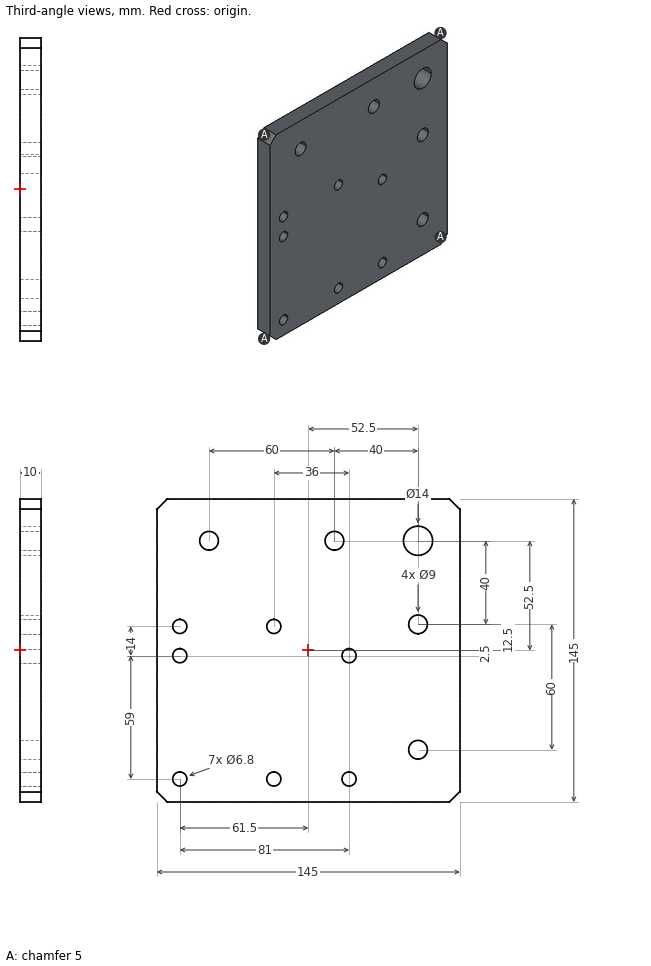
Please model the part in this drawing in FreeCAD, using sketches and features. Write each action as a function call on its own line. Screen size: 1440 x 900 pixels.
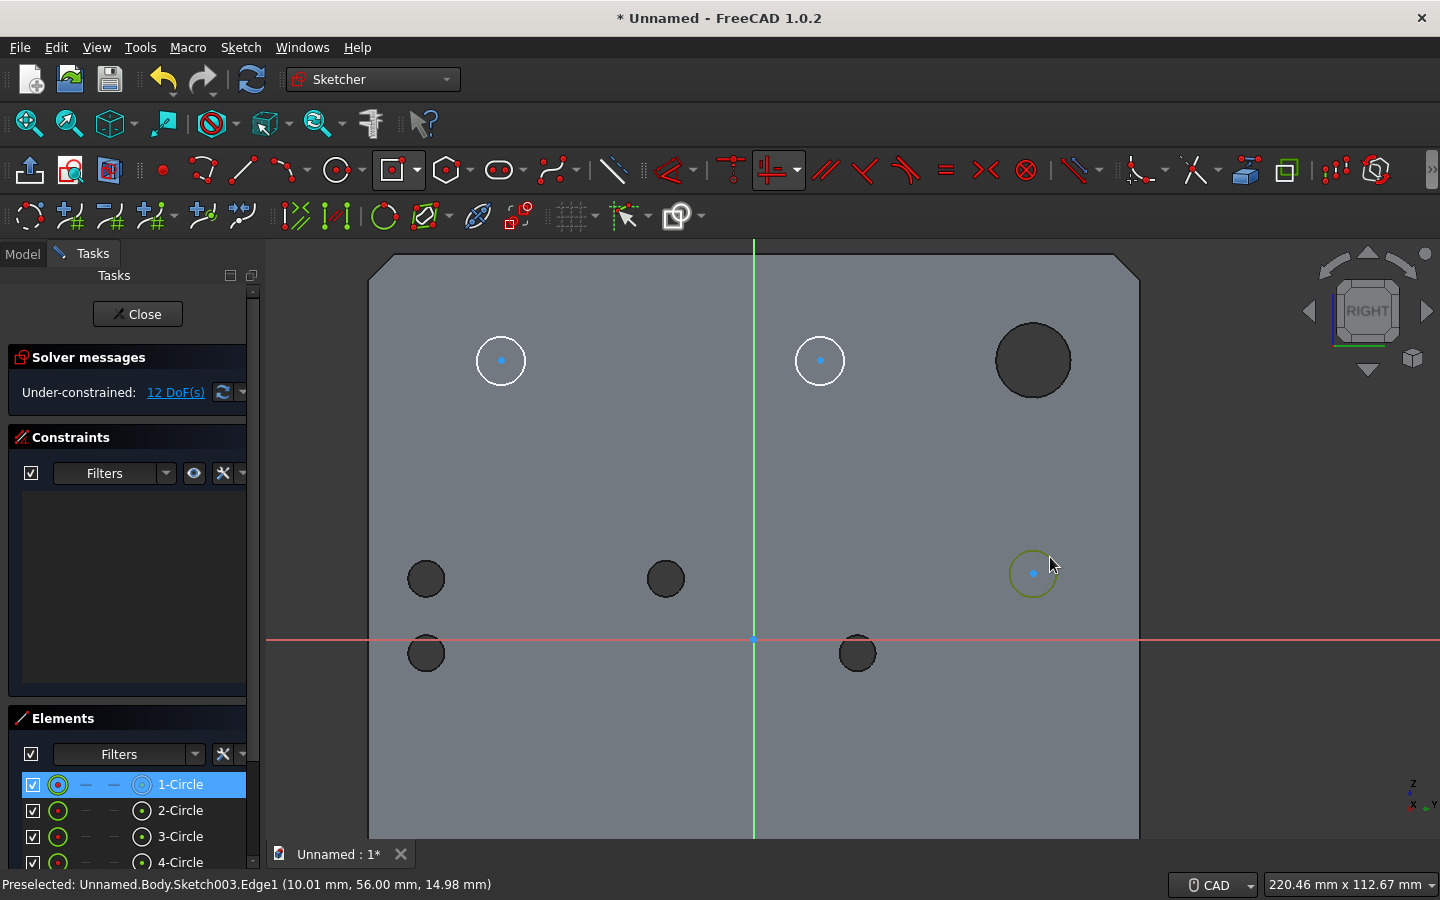
scroll(820, 361, down, 2)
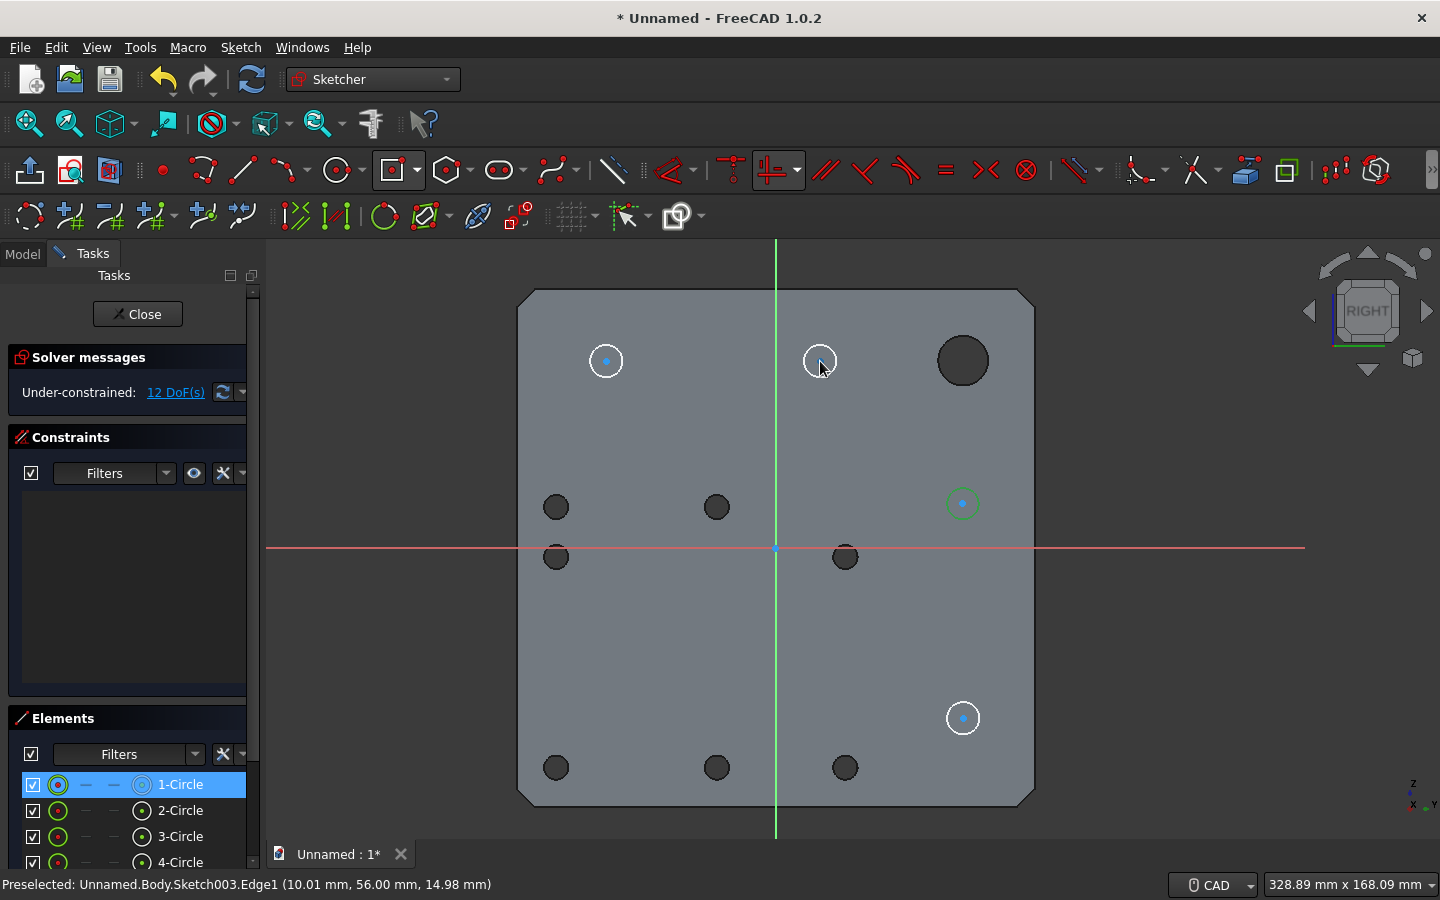
click(975, 707)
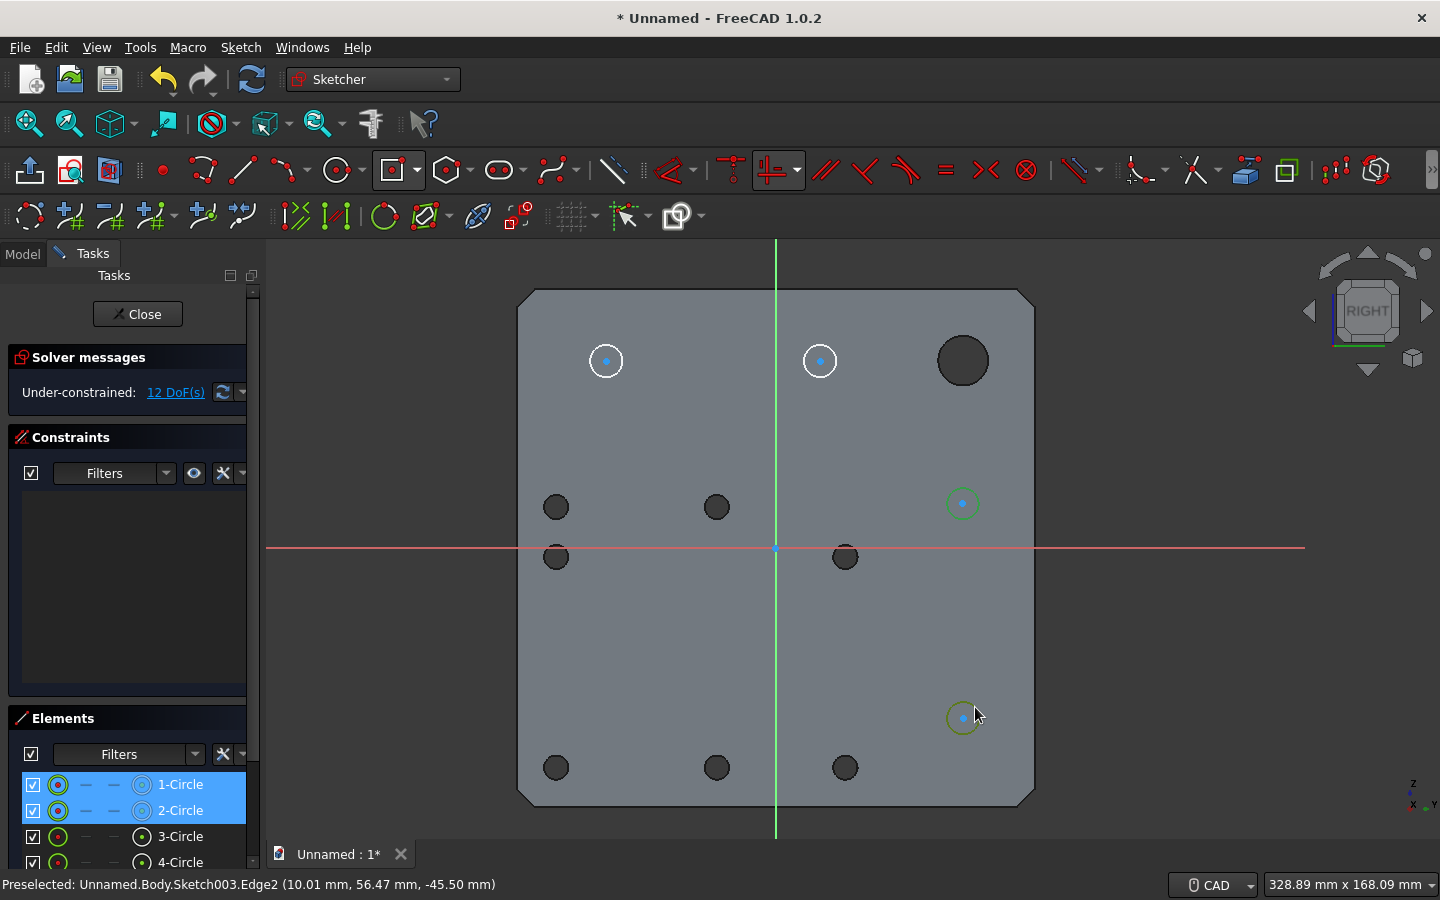
click(832, 350)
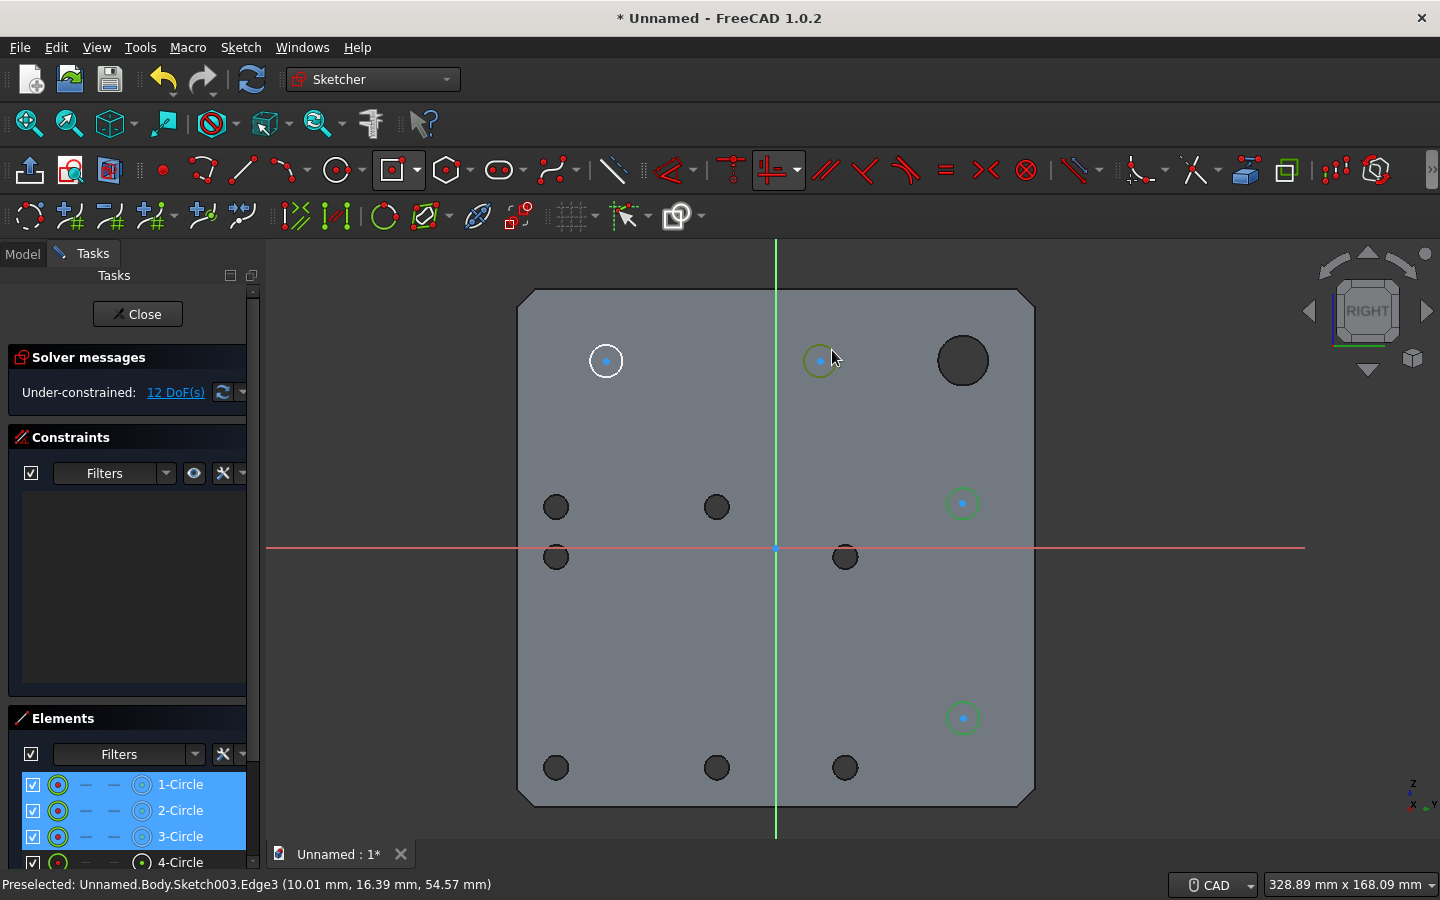
click(618, 350)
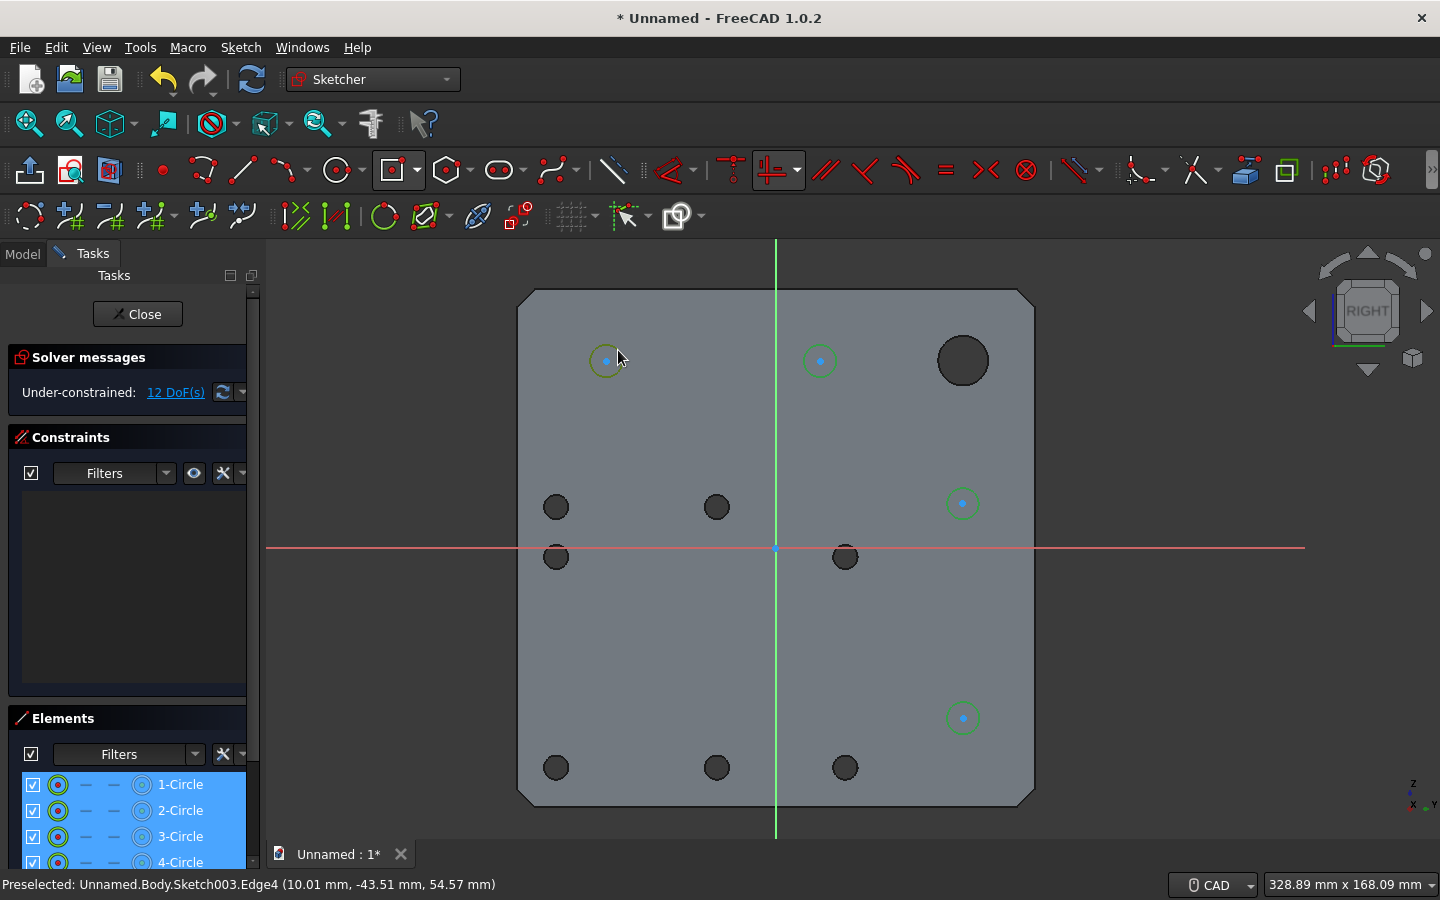
key(e)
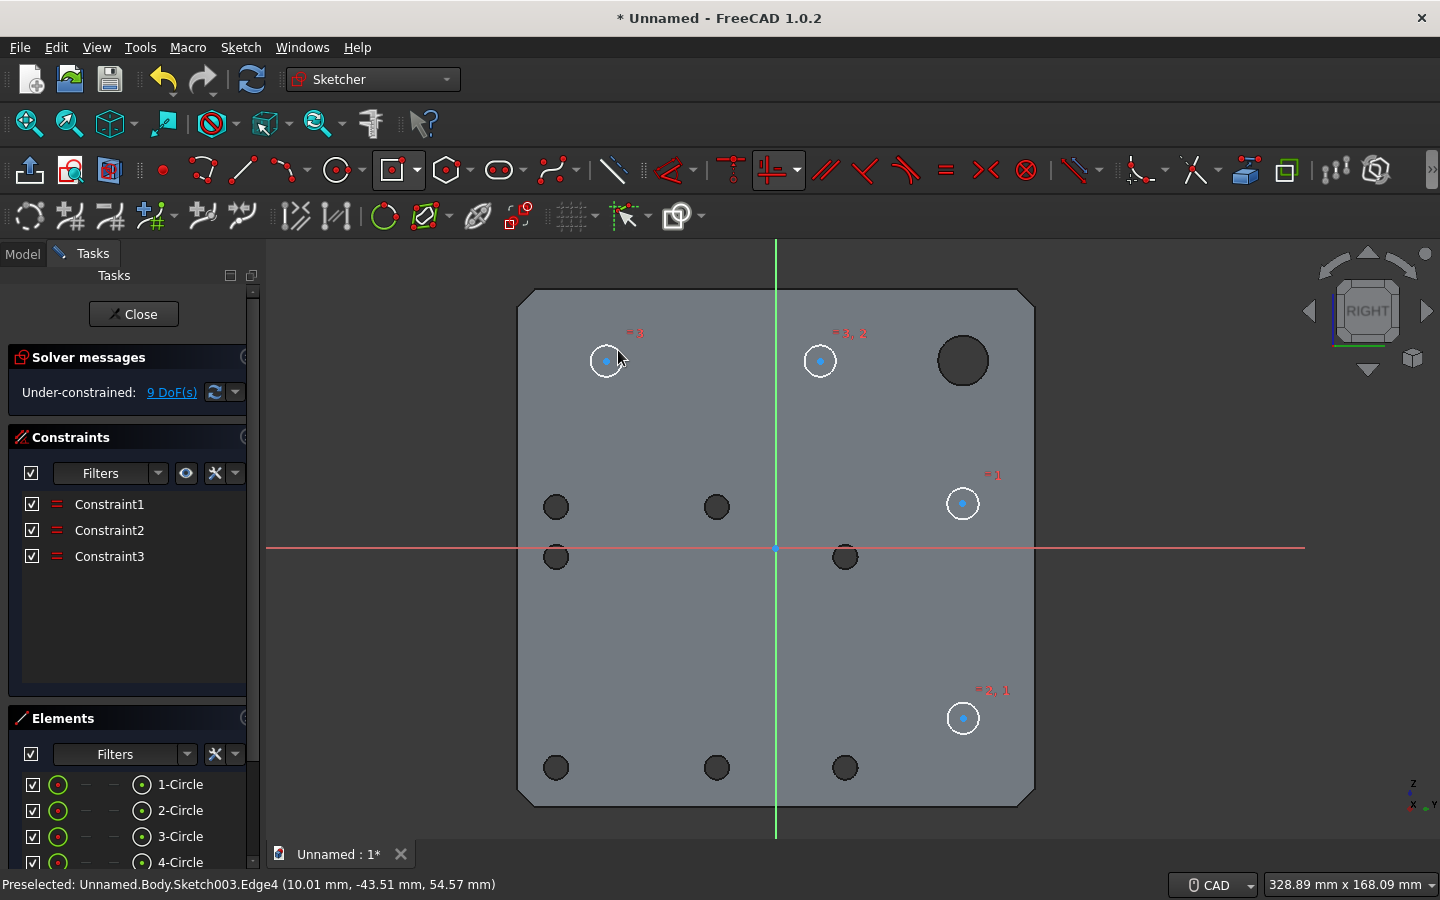
click(963, 504)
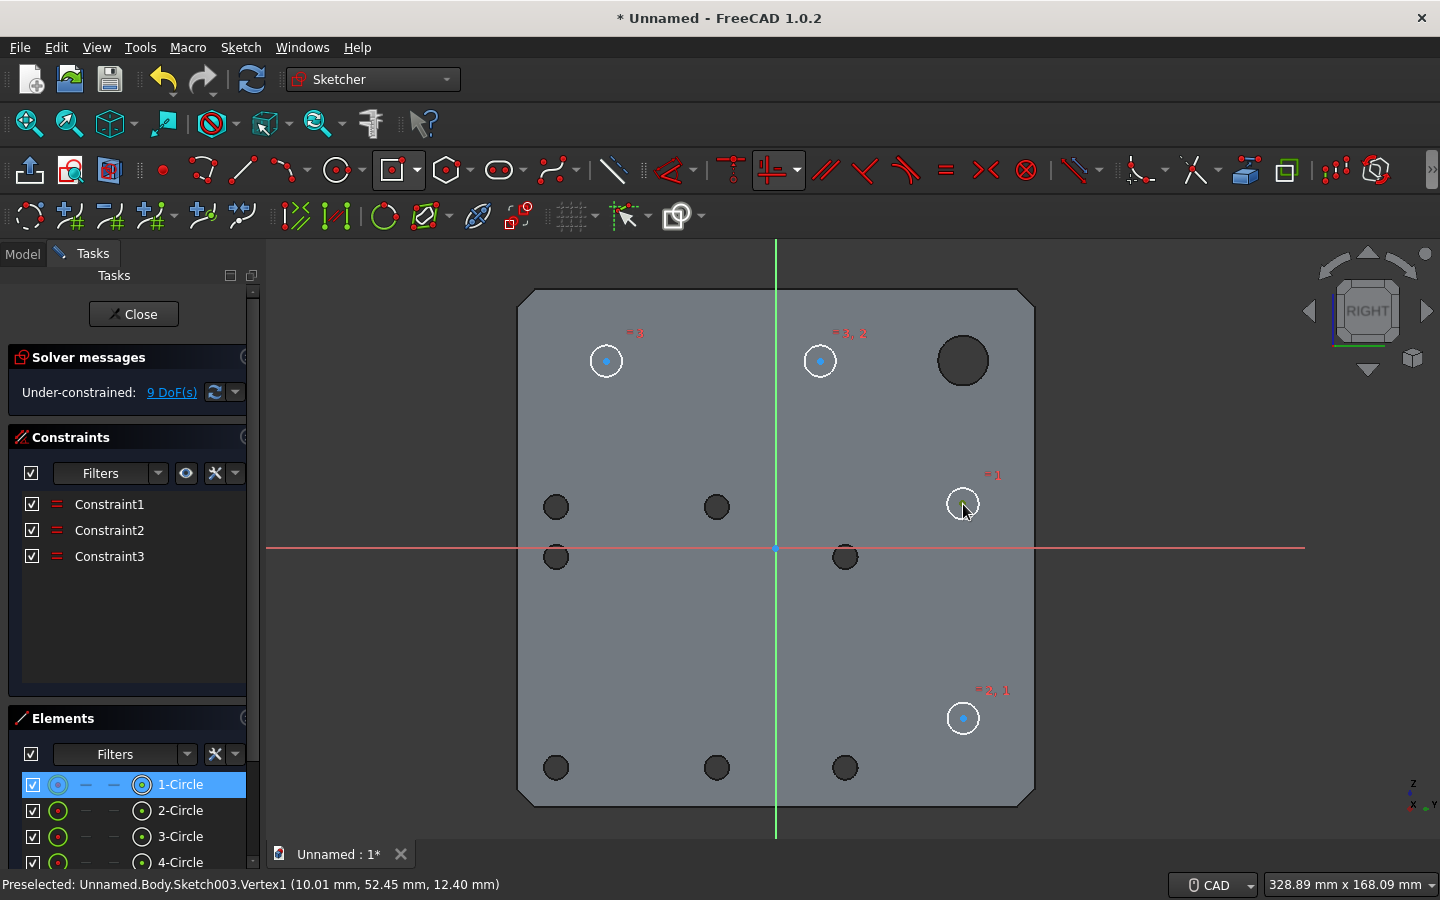
click(963, 718)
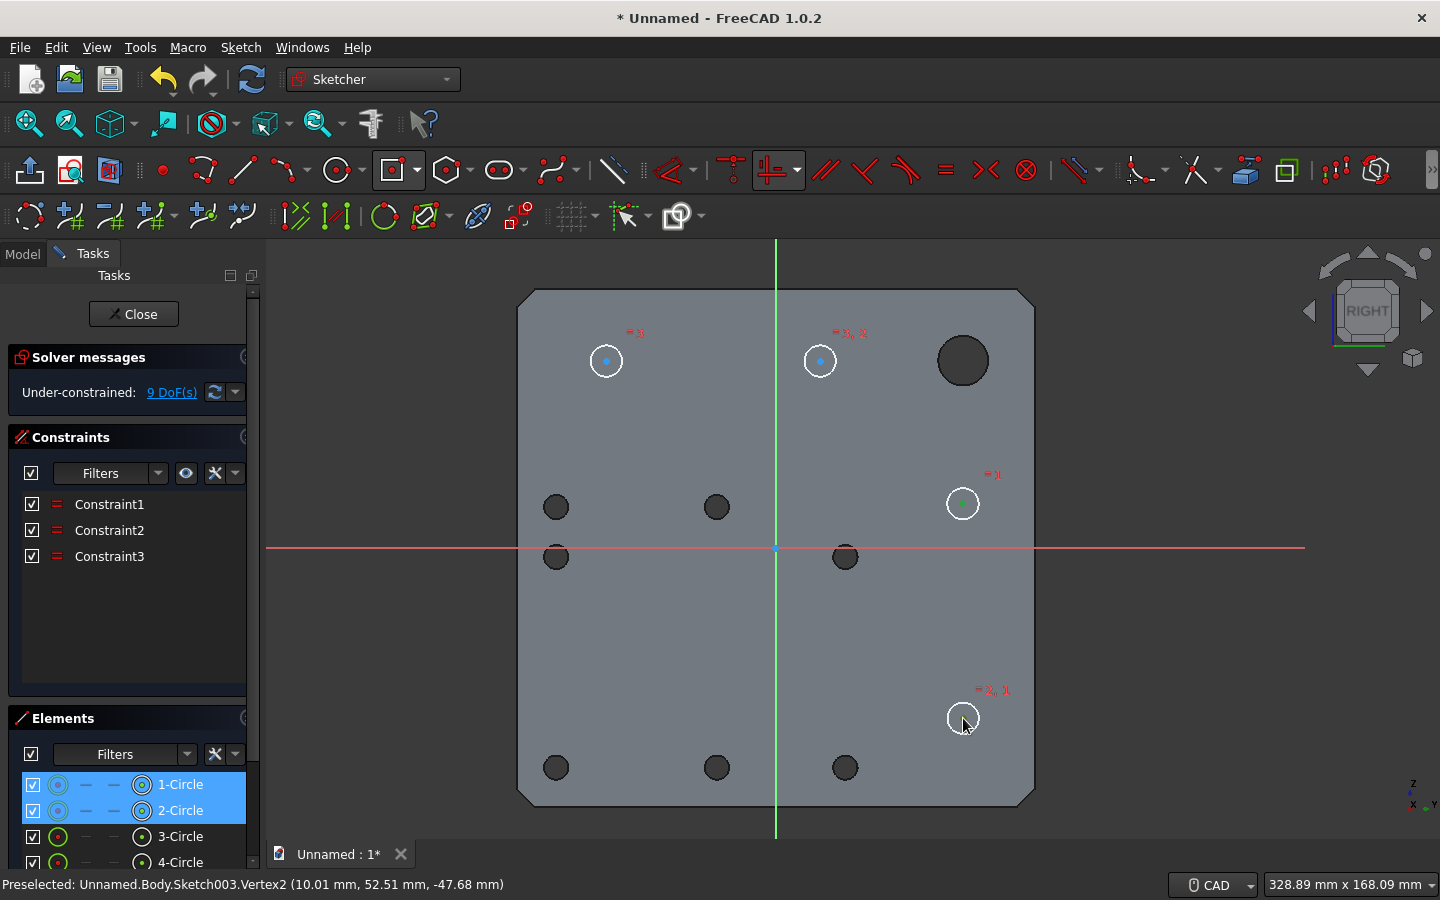
click(800, 170)